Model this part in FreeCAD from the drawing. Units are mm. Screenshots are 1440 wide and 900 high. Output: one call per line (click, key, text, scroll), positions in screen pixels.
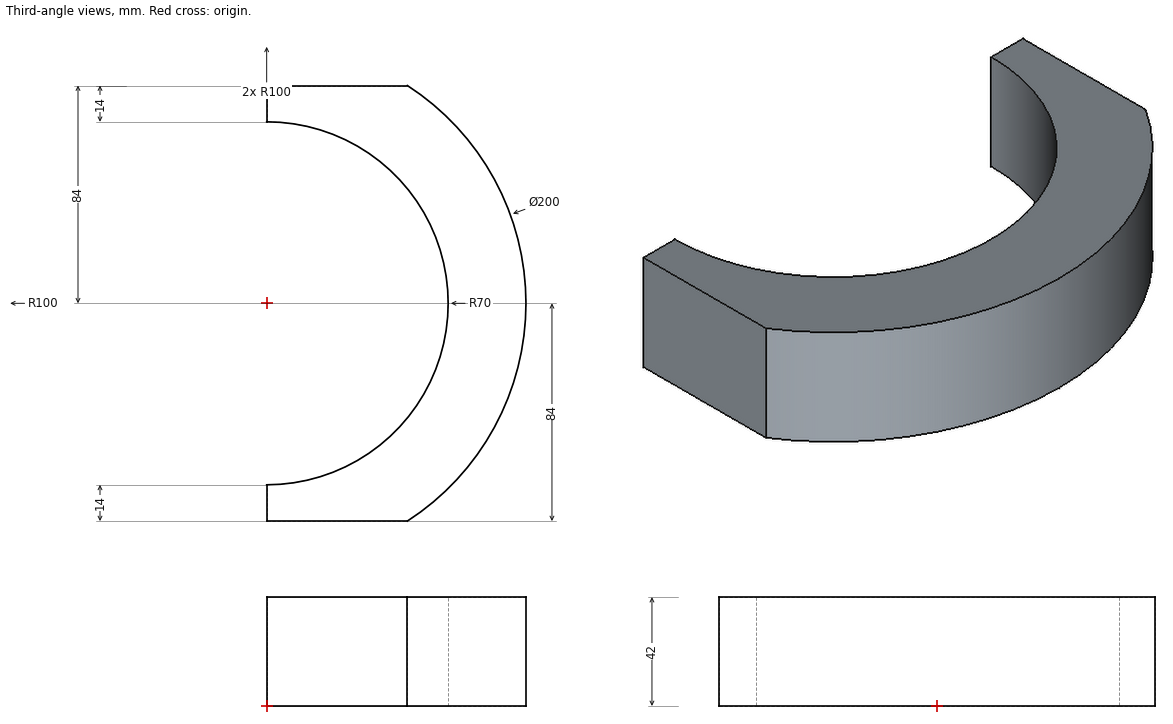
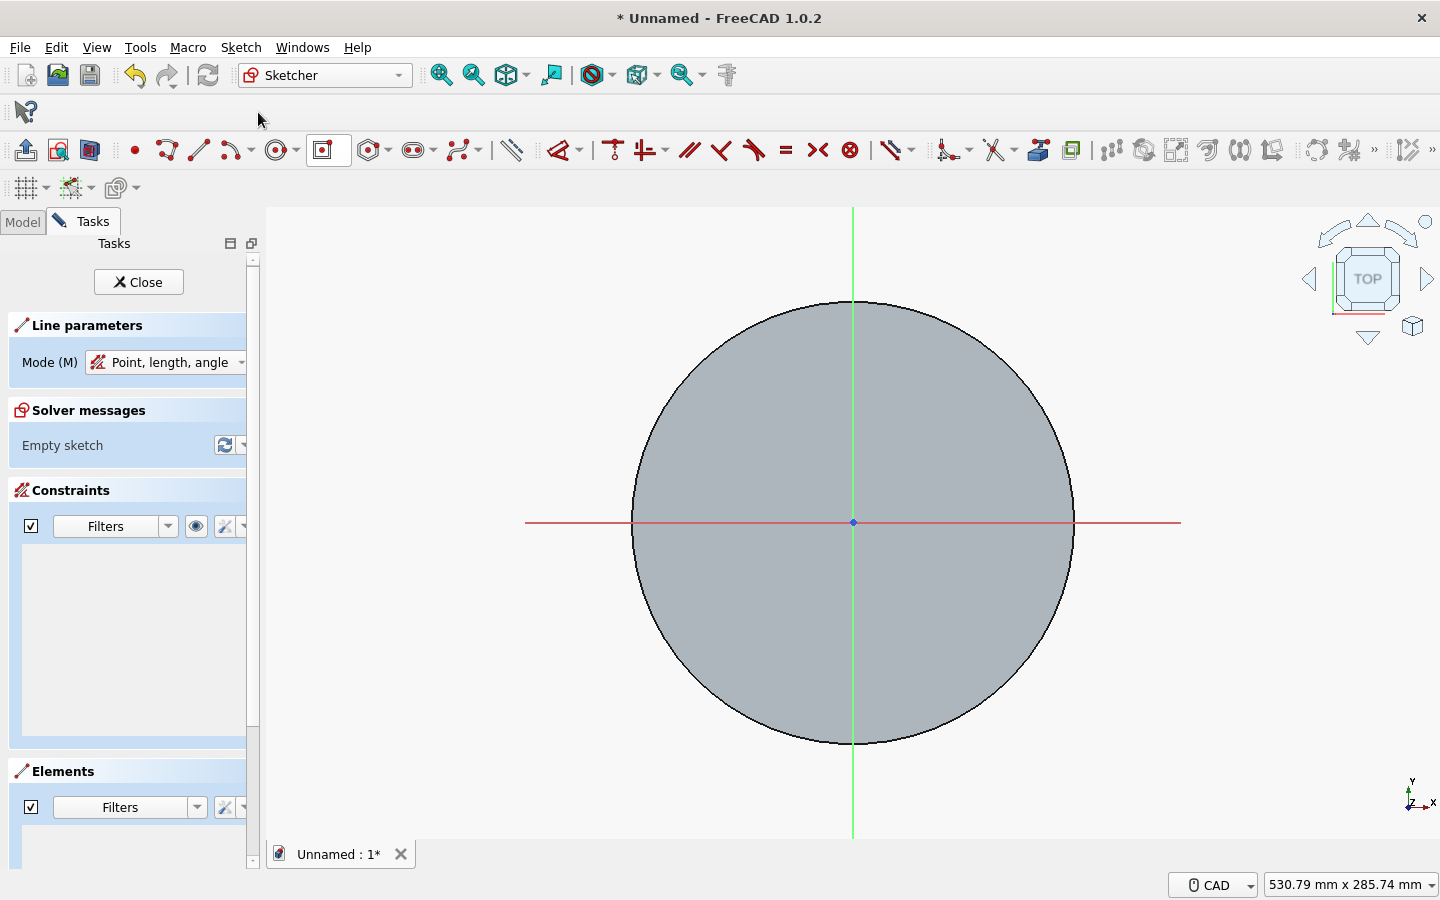
click(733, 337)
click(973, 337)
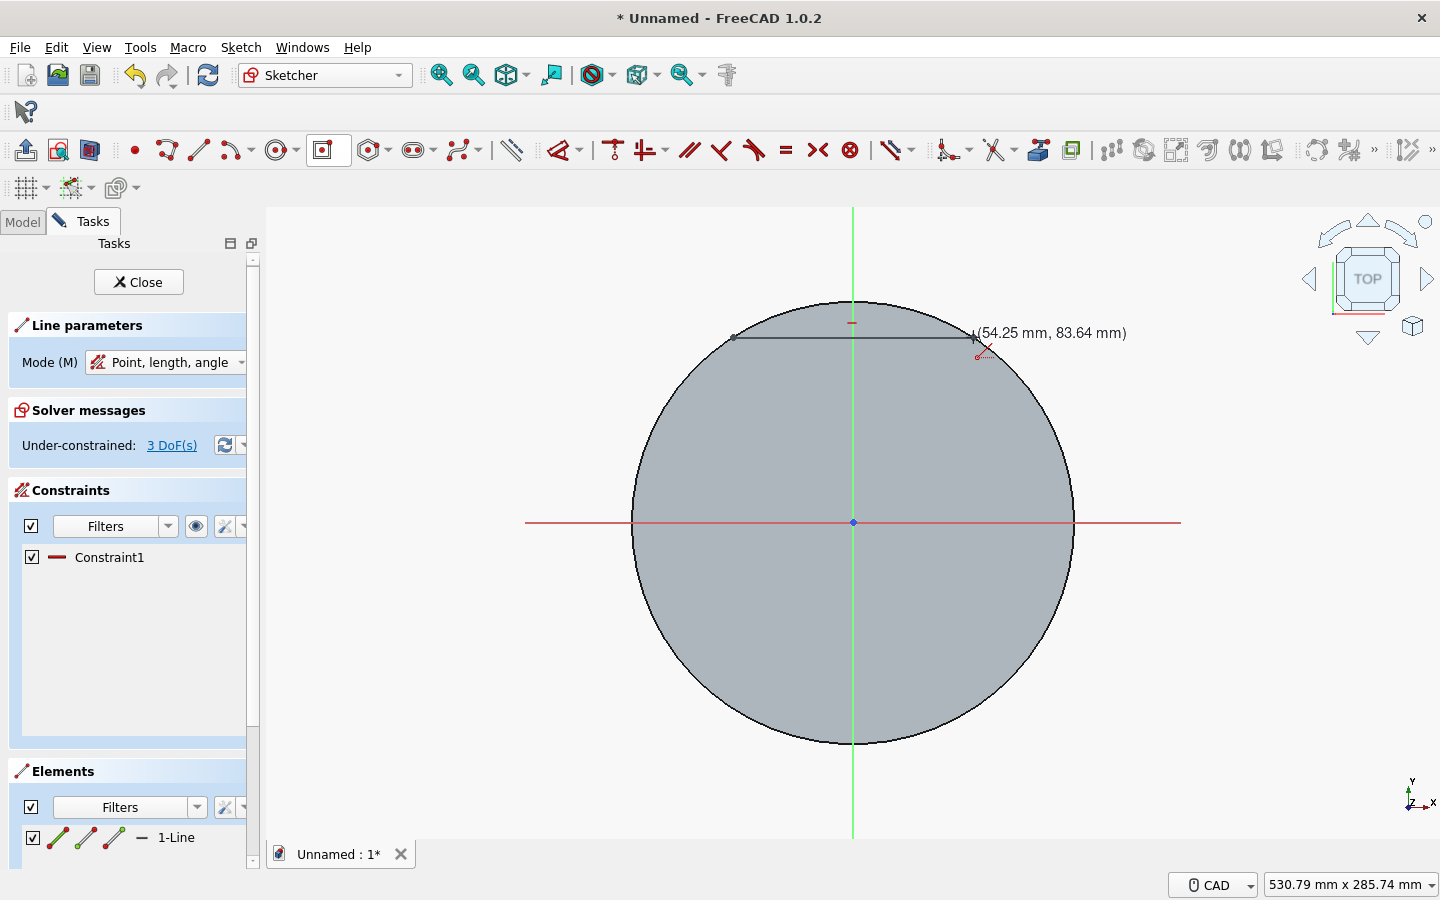
key(g)
key(3)
key(a)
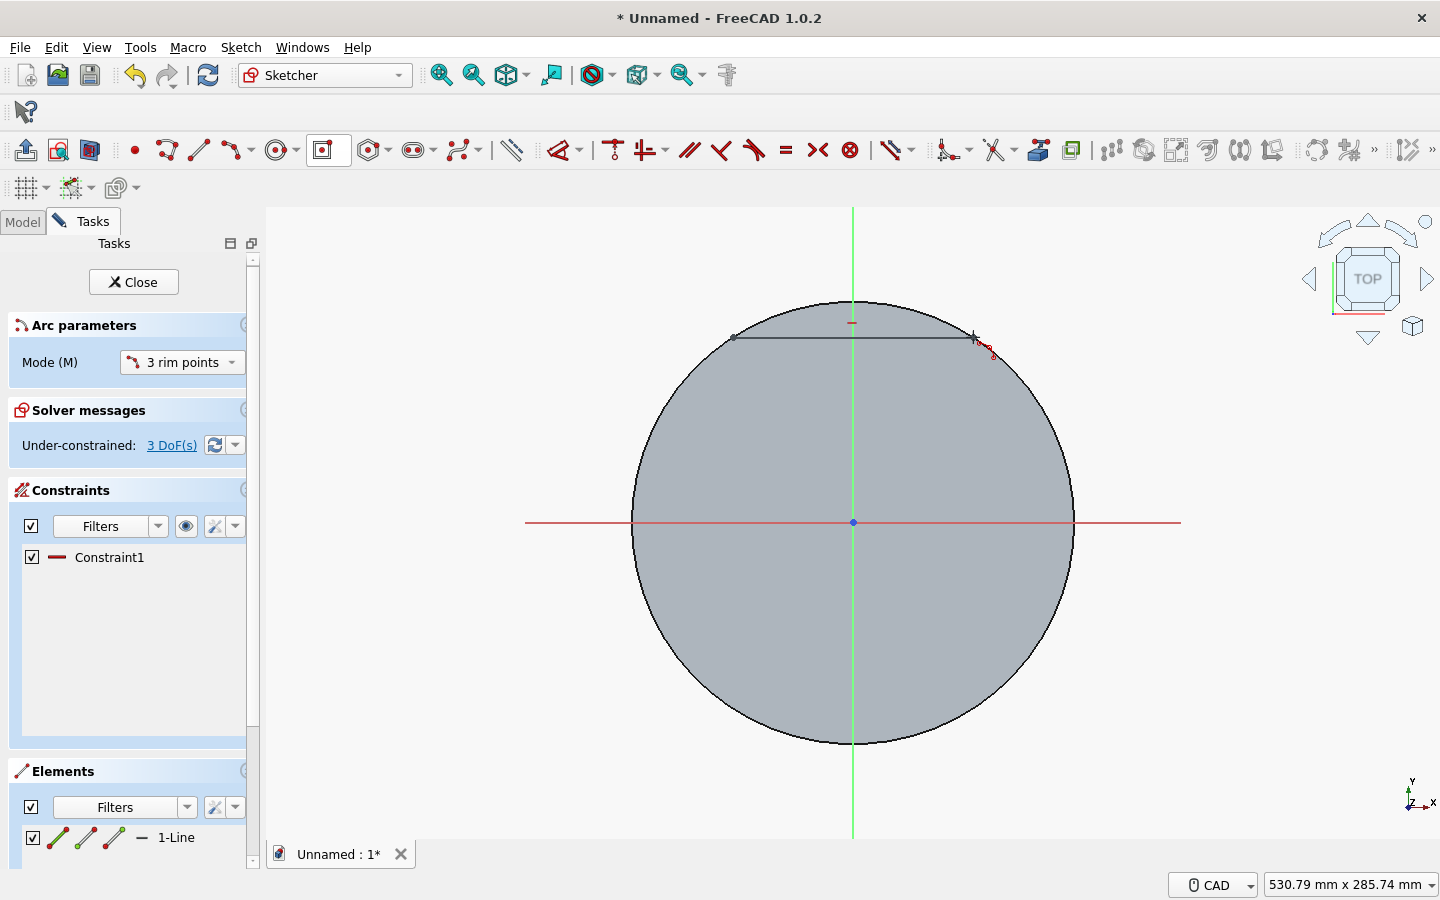
click(973, 338)
click(733, 338)
click(878, 303)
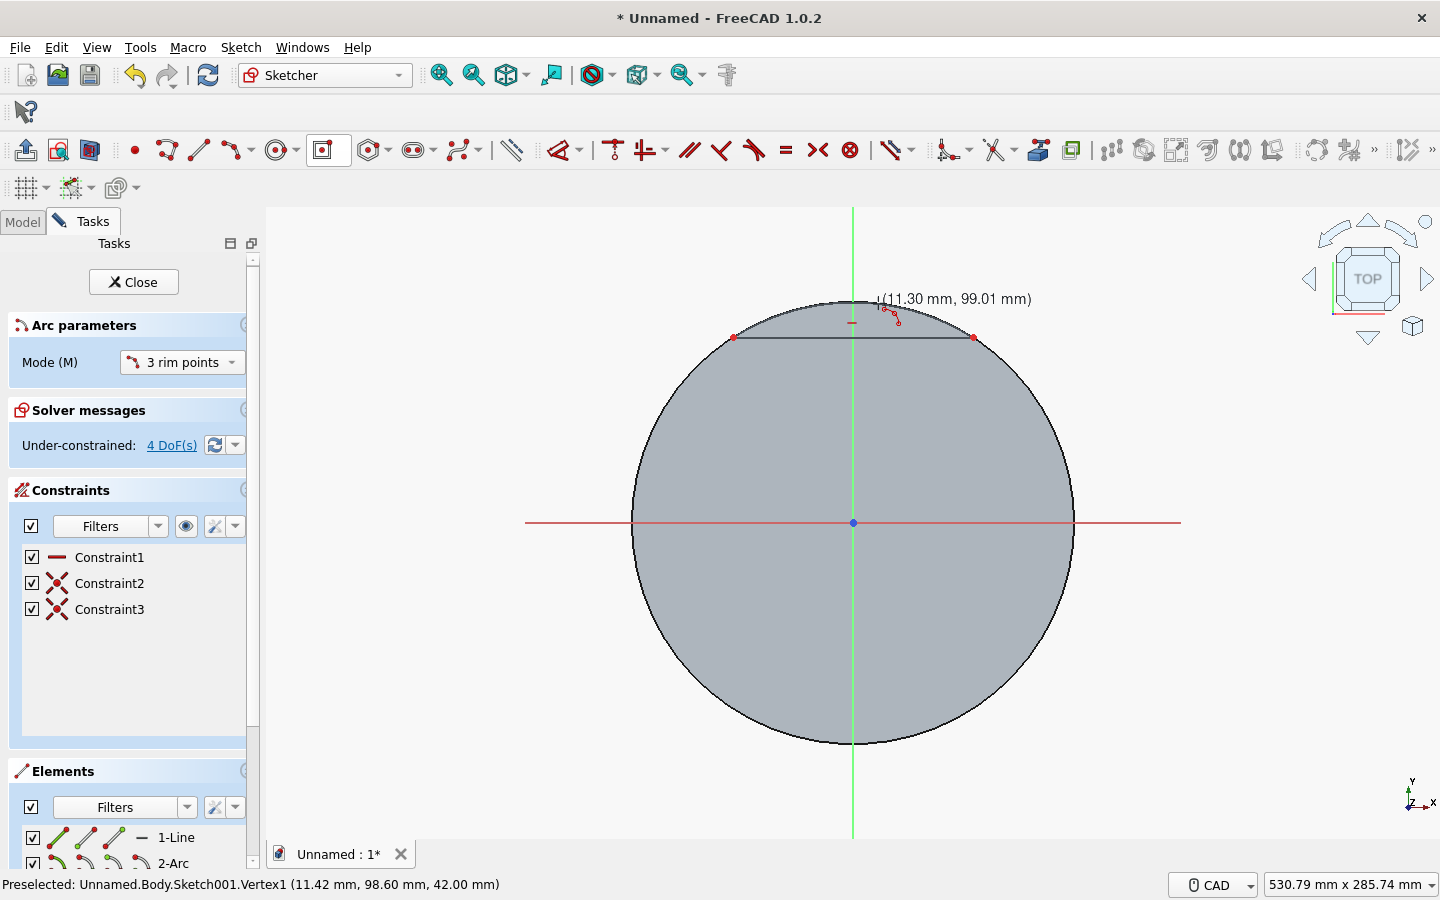
click(200, 150)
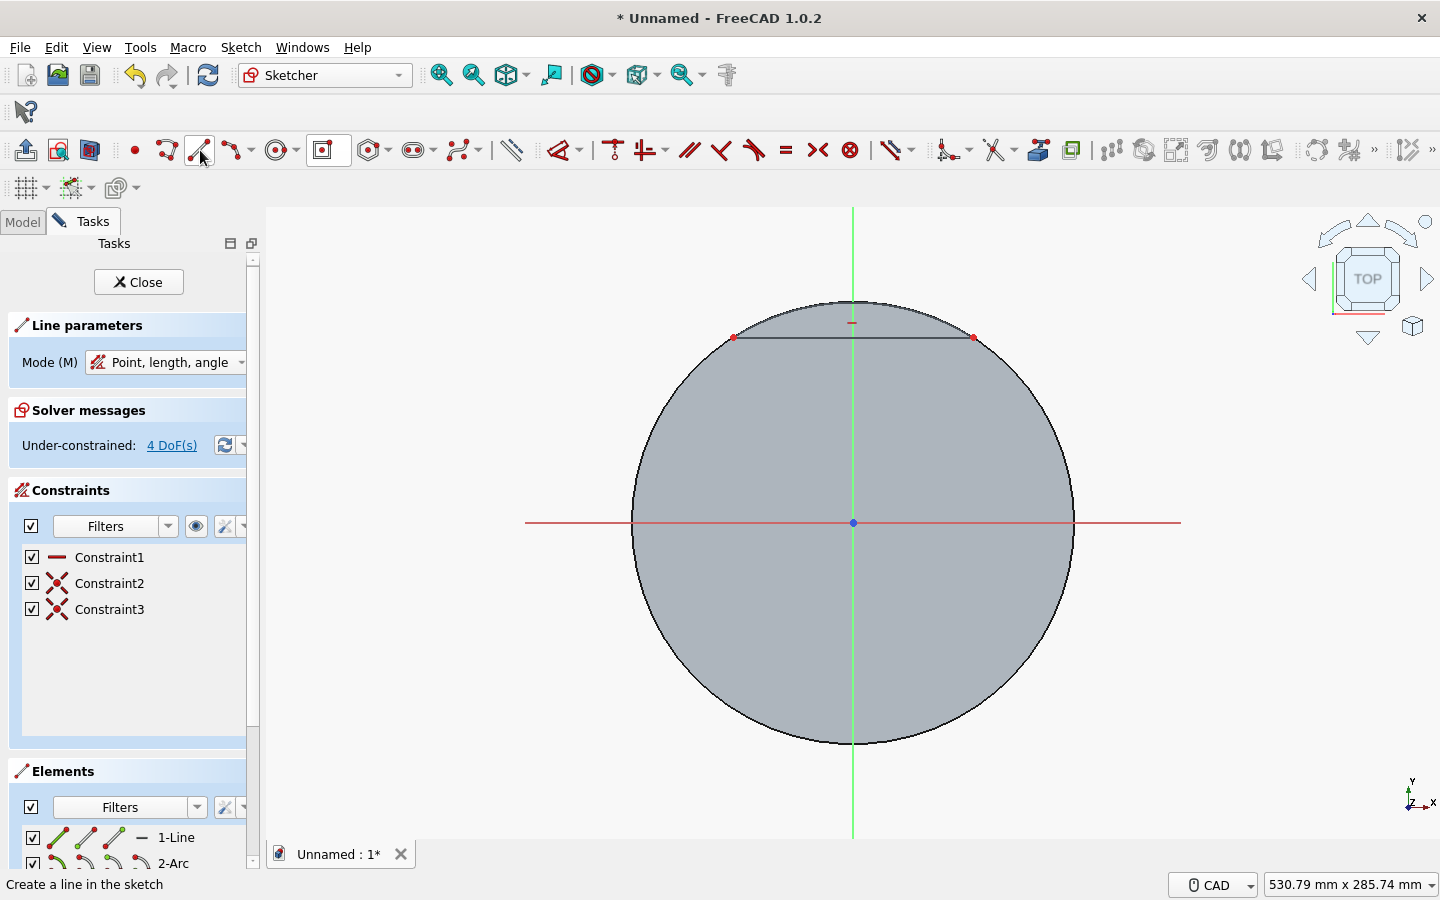
click(973, 709)
click(733, 709)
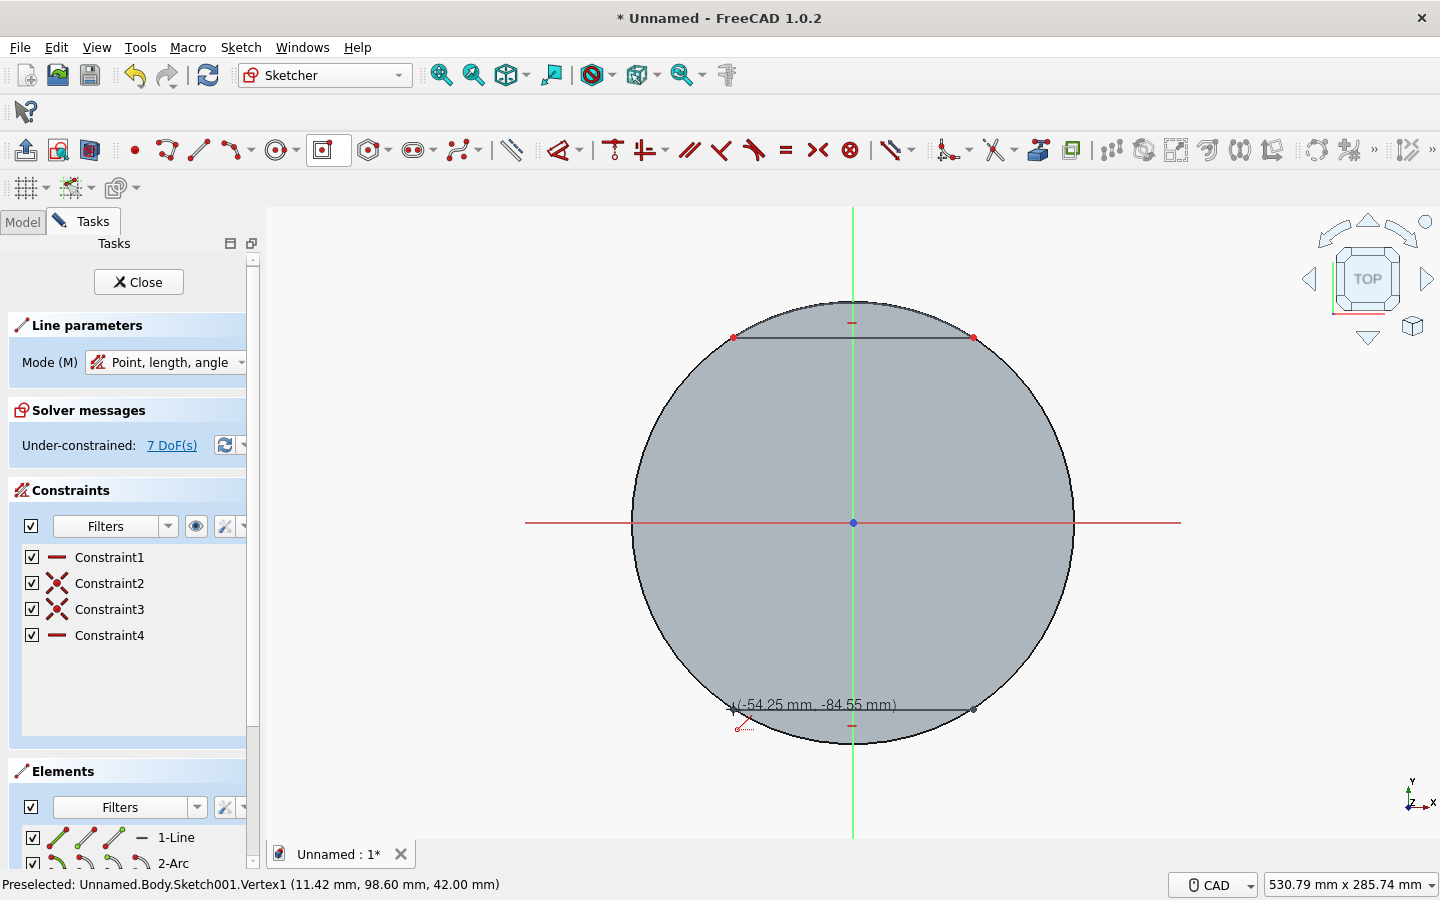
click(232, 150)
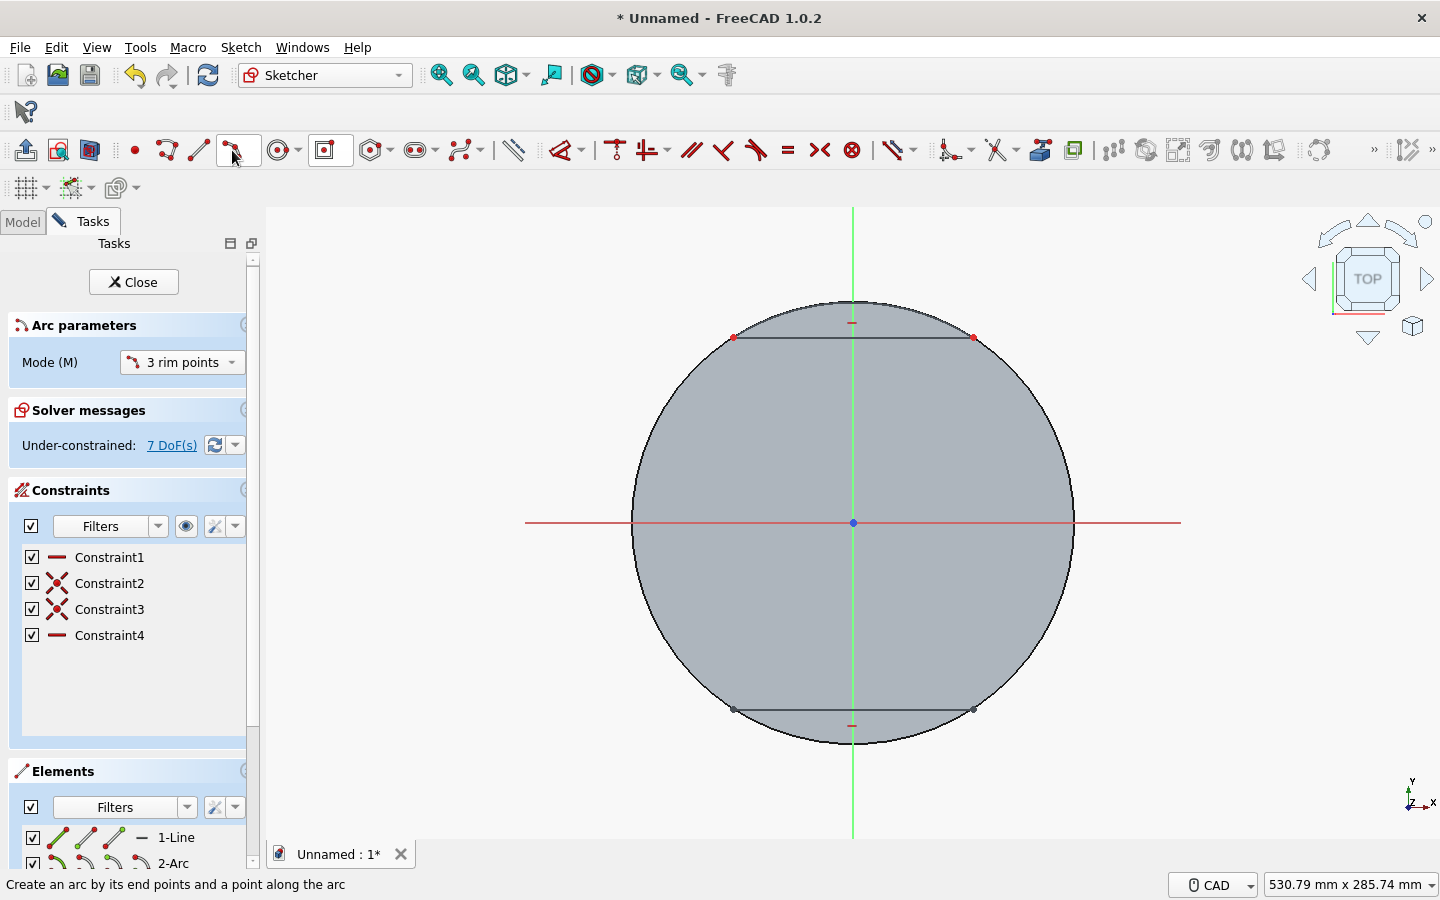
click(733, 710)
click(973, 710)
click(828, 743)
key(Escape)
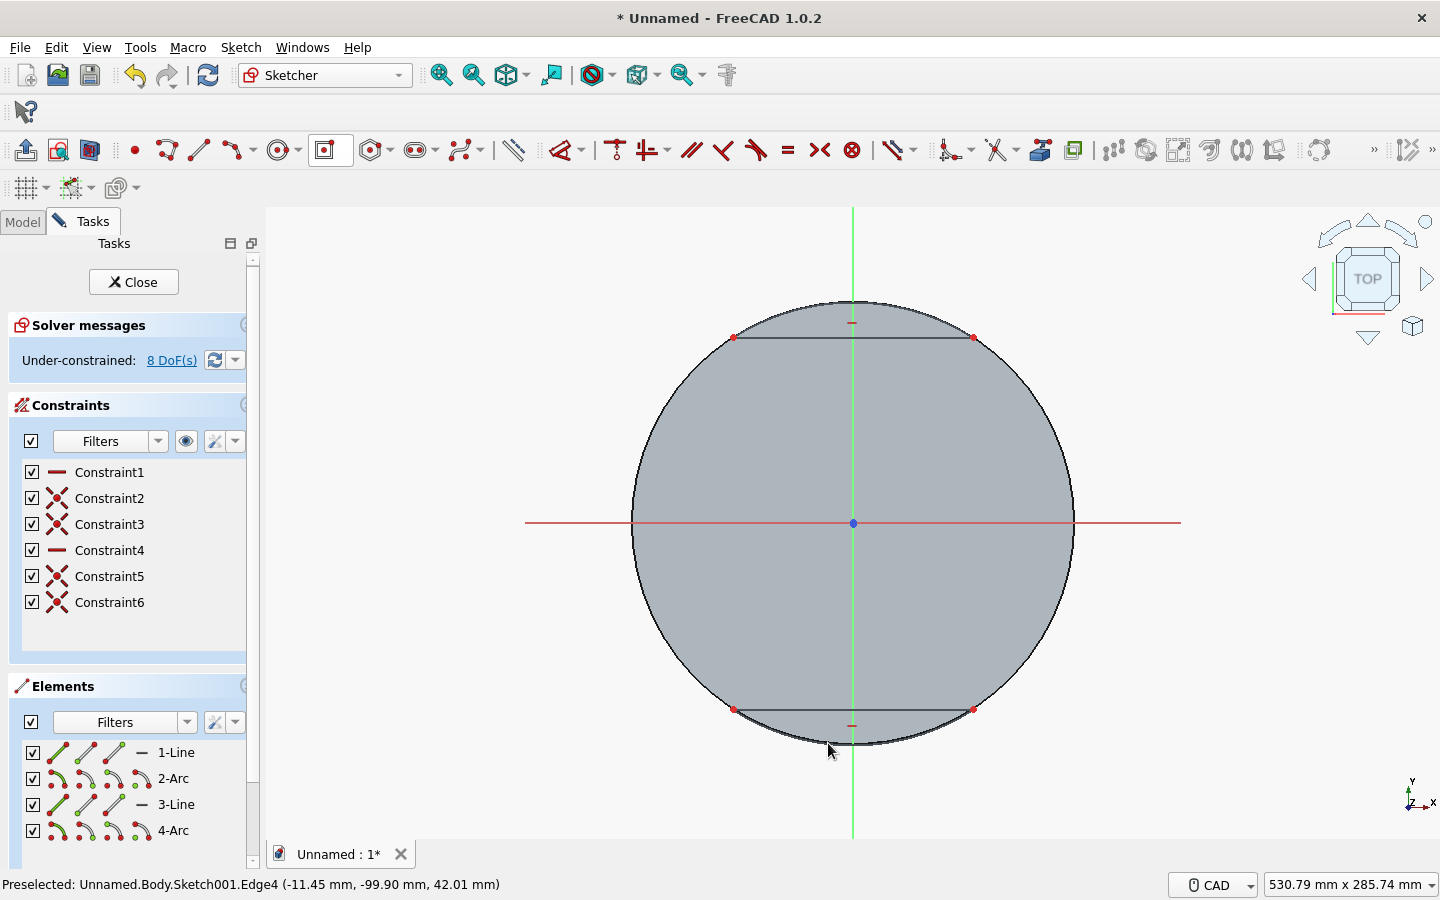
click(903, 308)